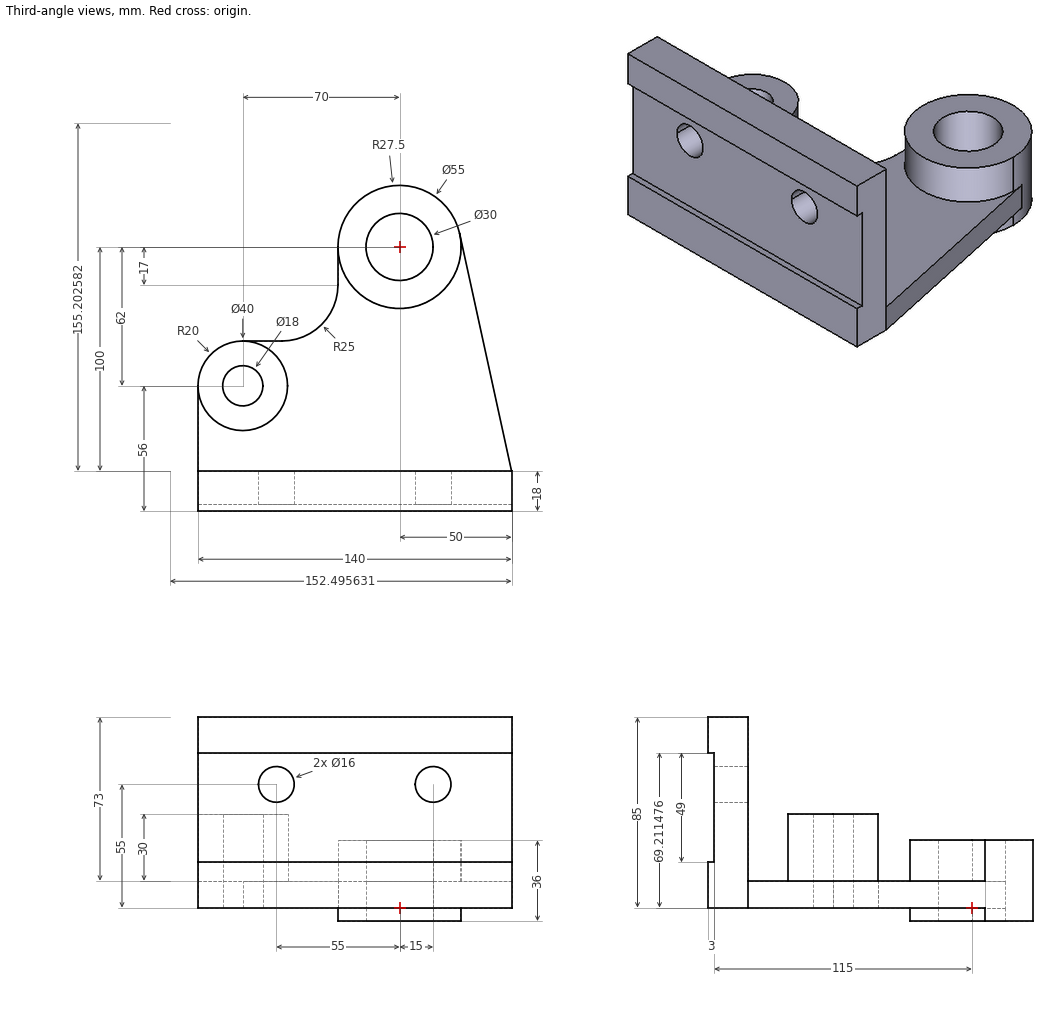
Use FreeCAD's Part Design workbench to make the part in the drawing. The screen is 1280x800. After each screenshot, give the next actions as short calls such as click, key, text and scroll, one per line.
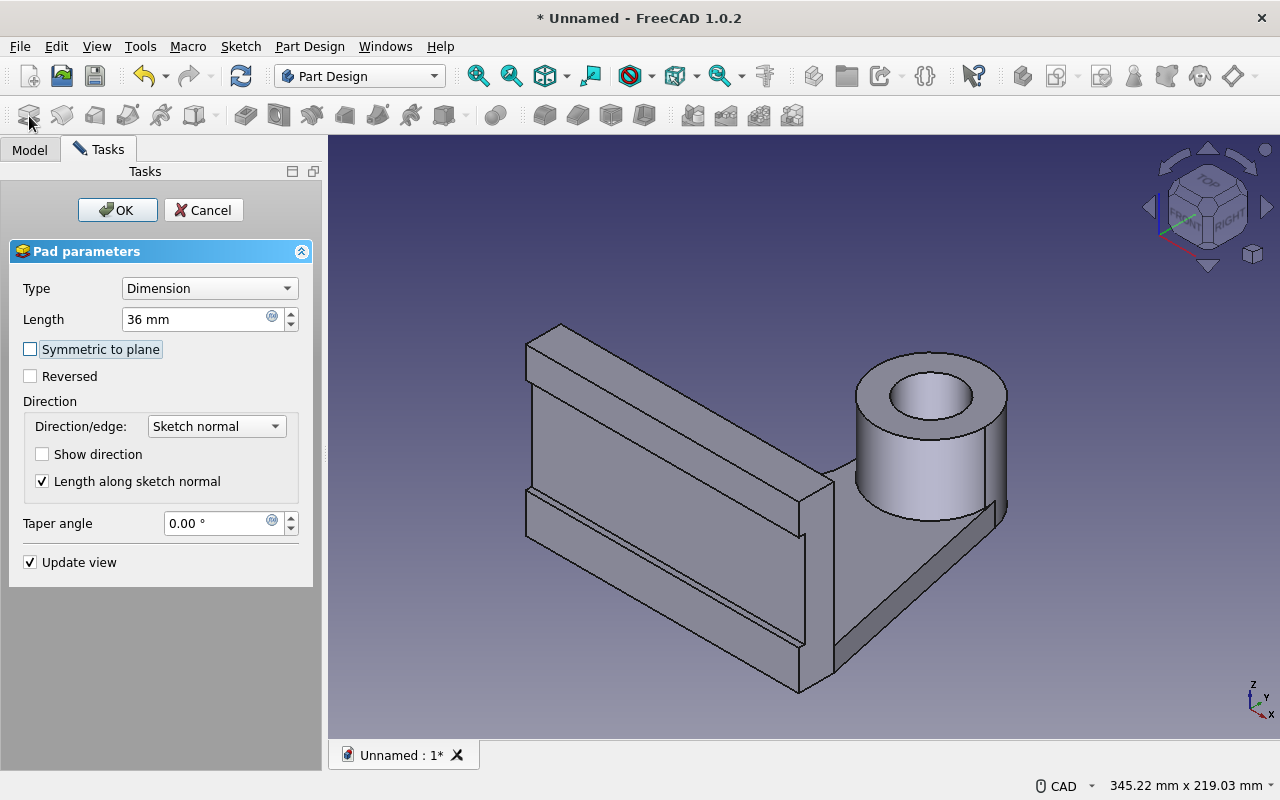
click(31, 349)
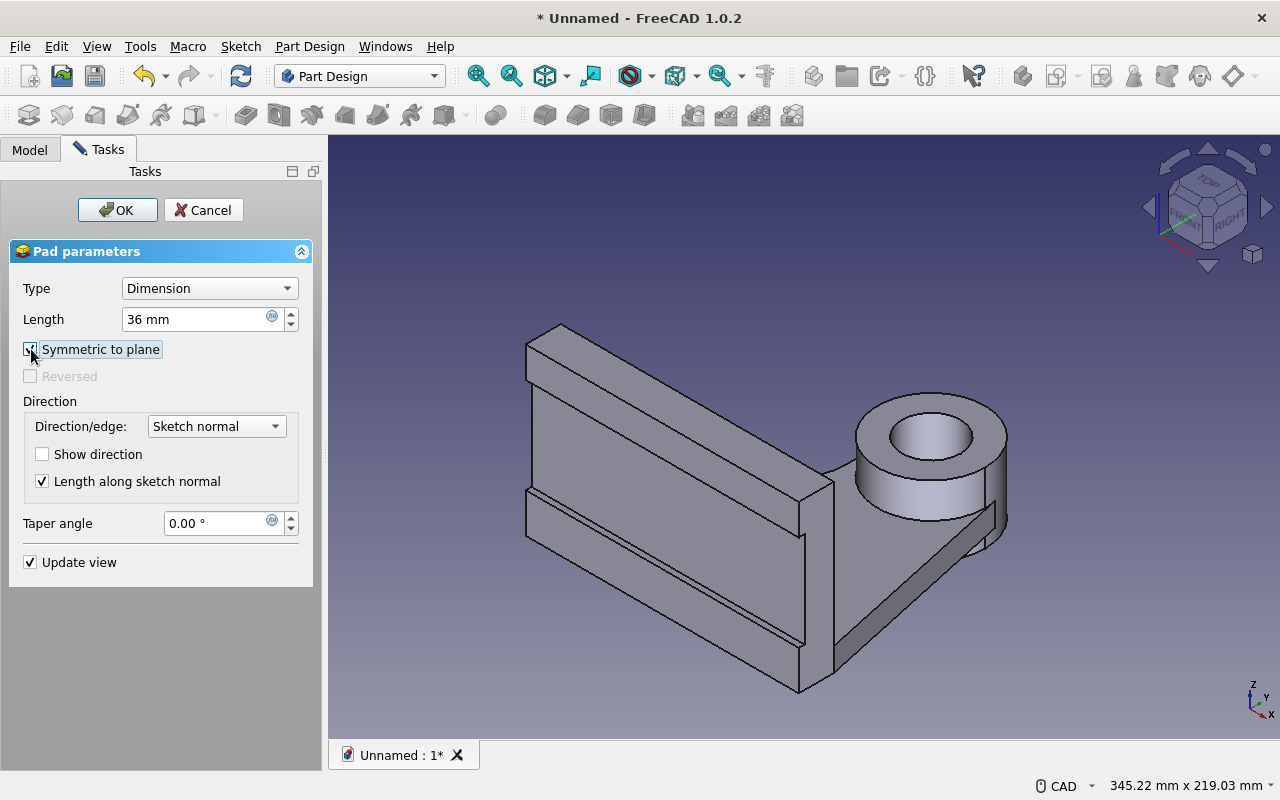
click(118, 210)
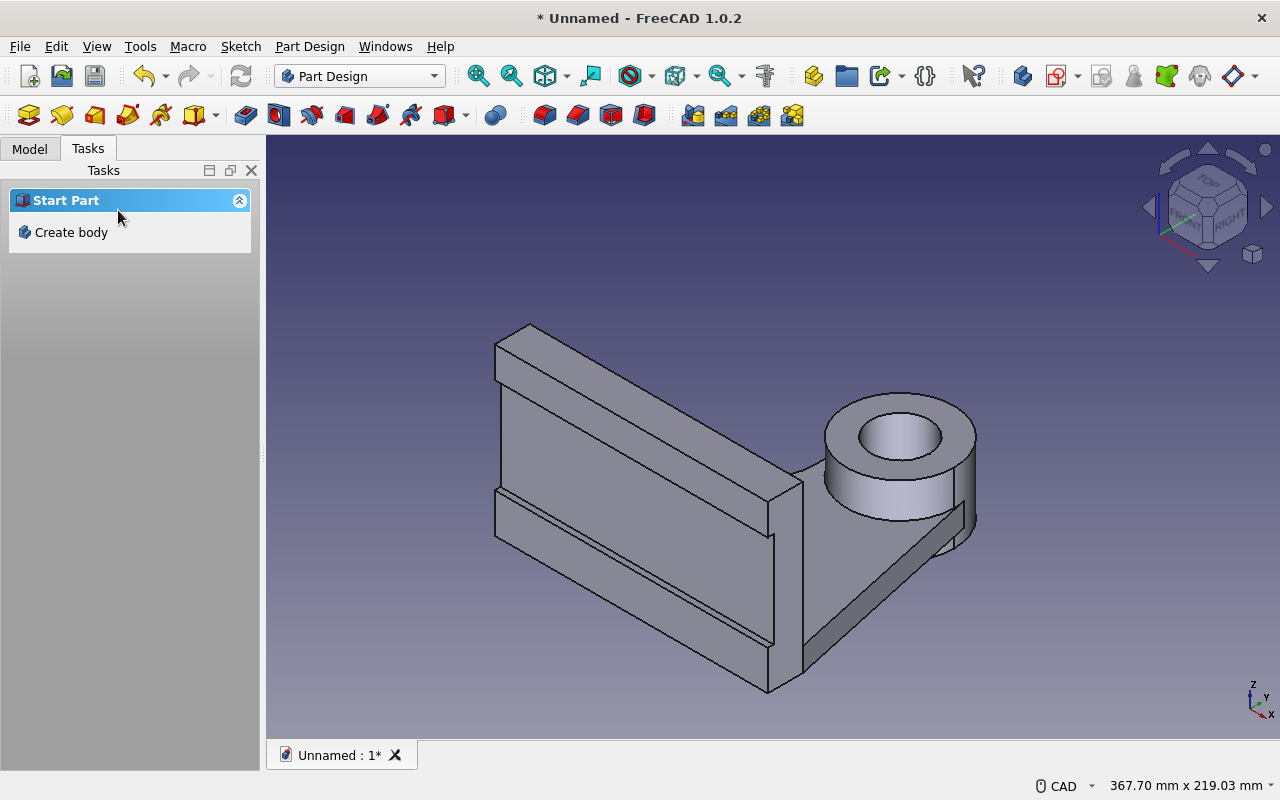
click(818, 569)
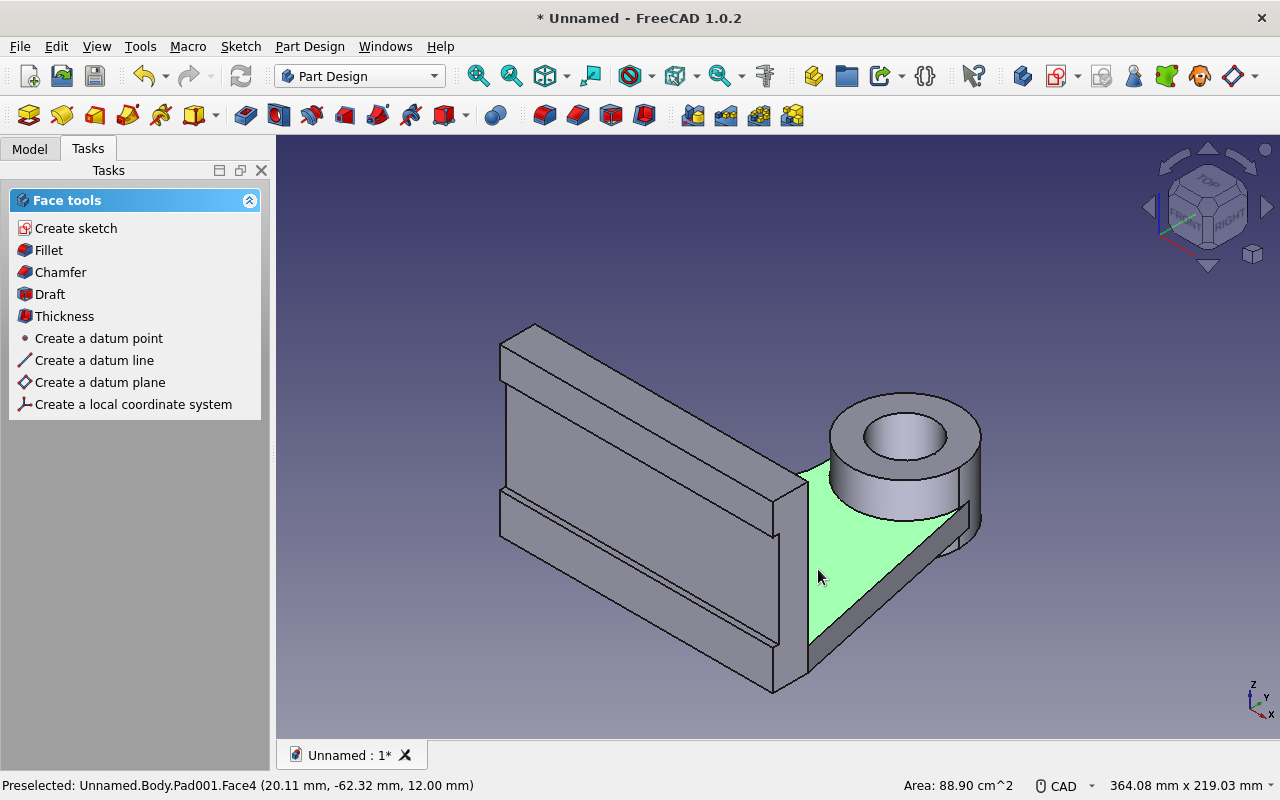
click(1056, 76)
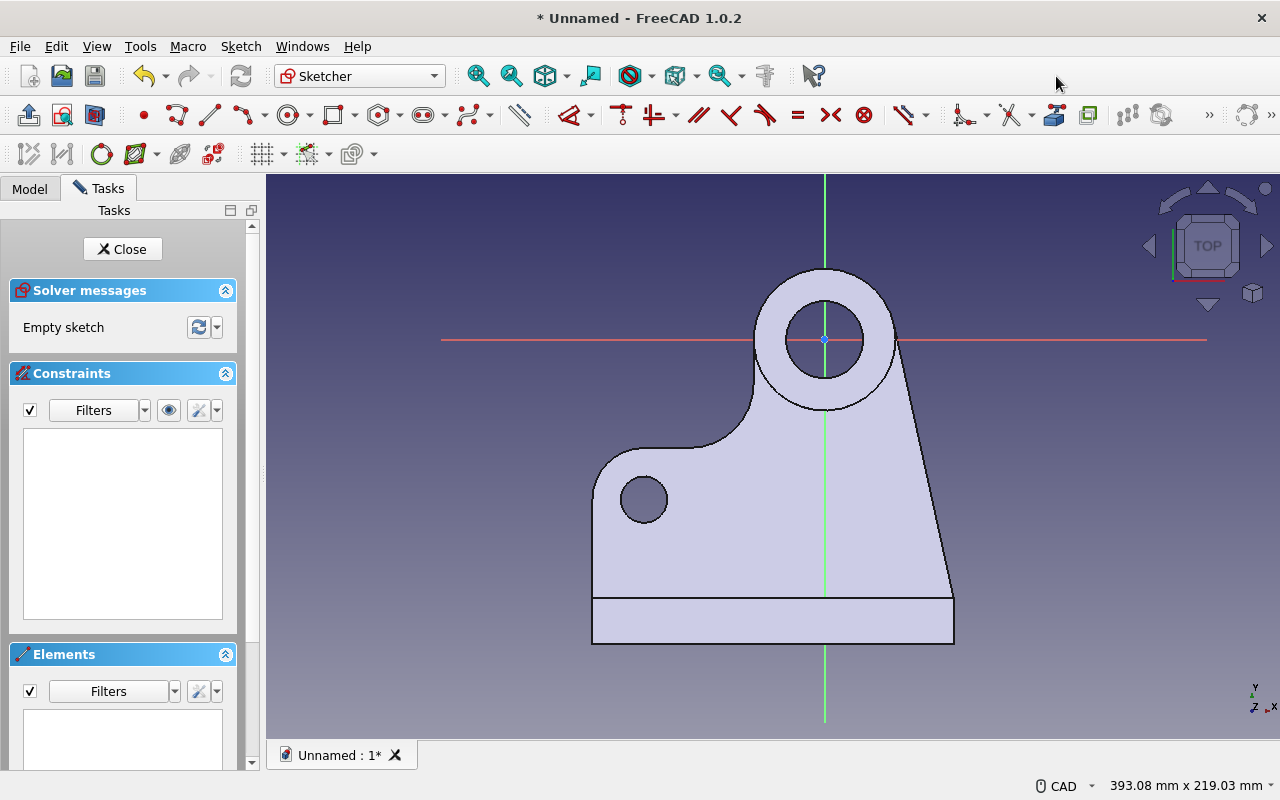
scroll(713, 432, up, 3)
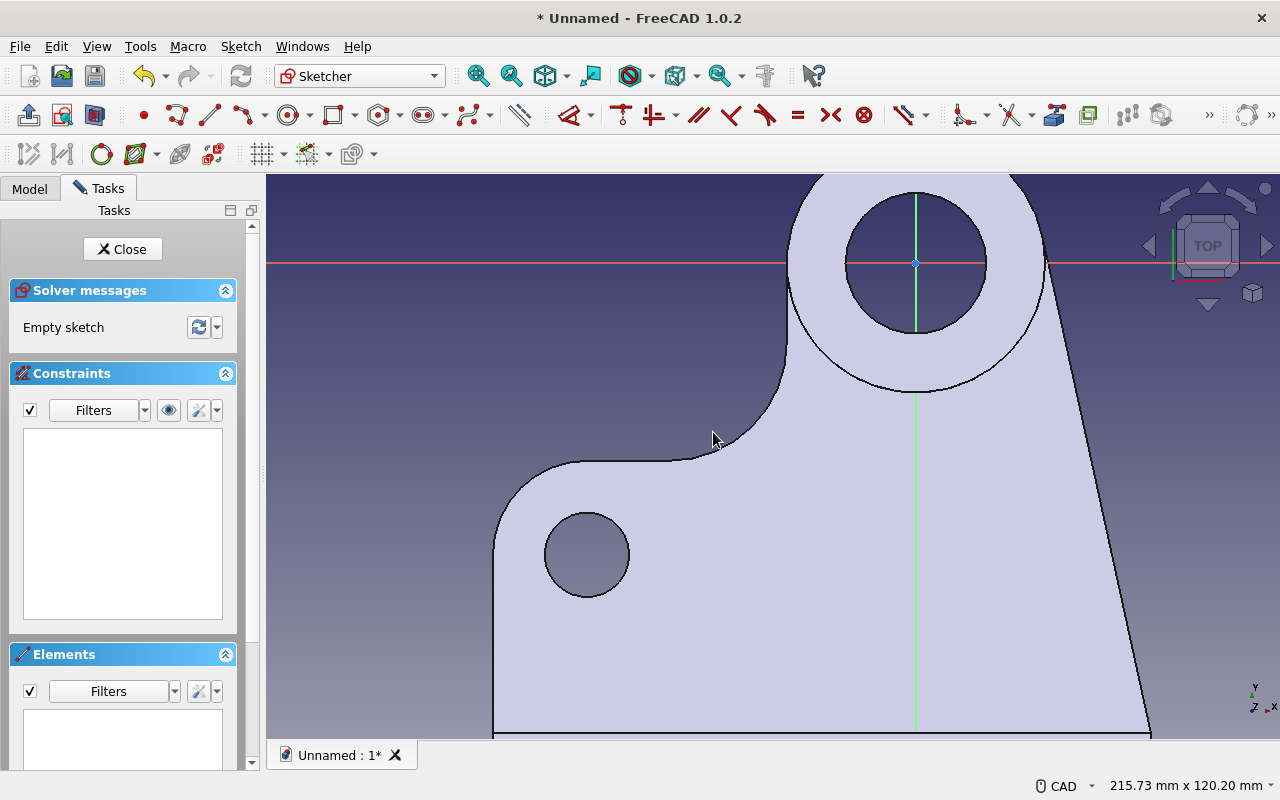
click(288, 116)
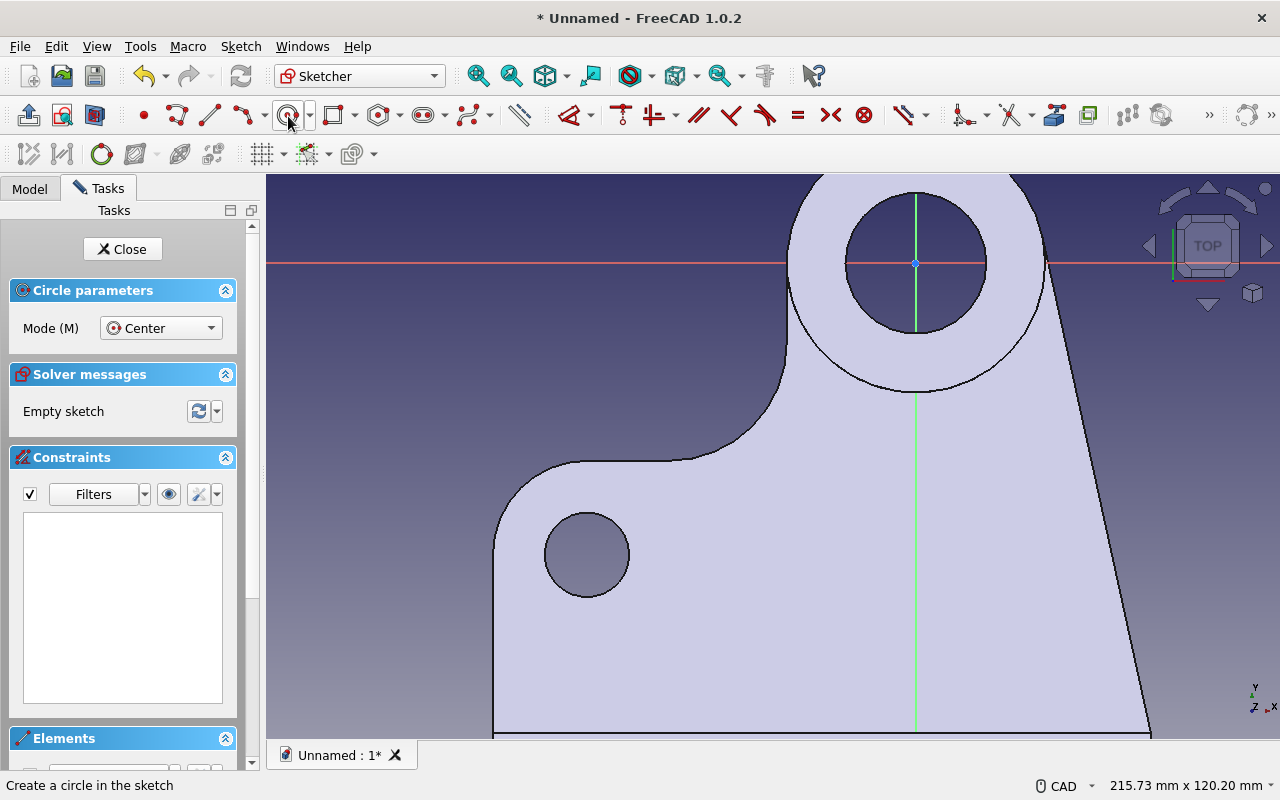
click(587, 555)
click(653, 488)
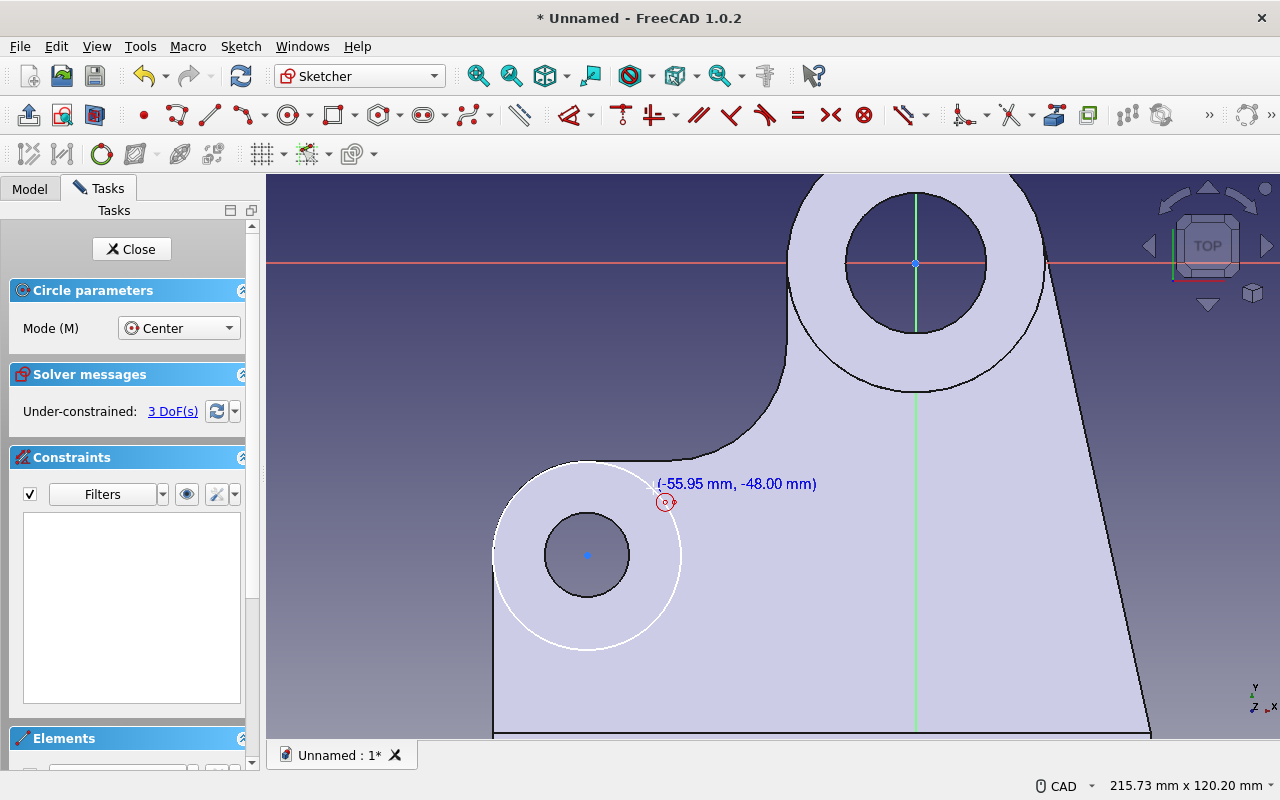
click(587, 556)
click(617, 525)
key(Escape)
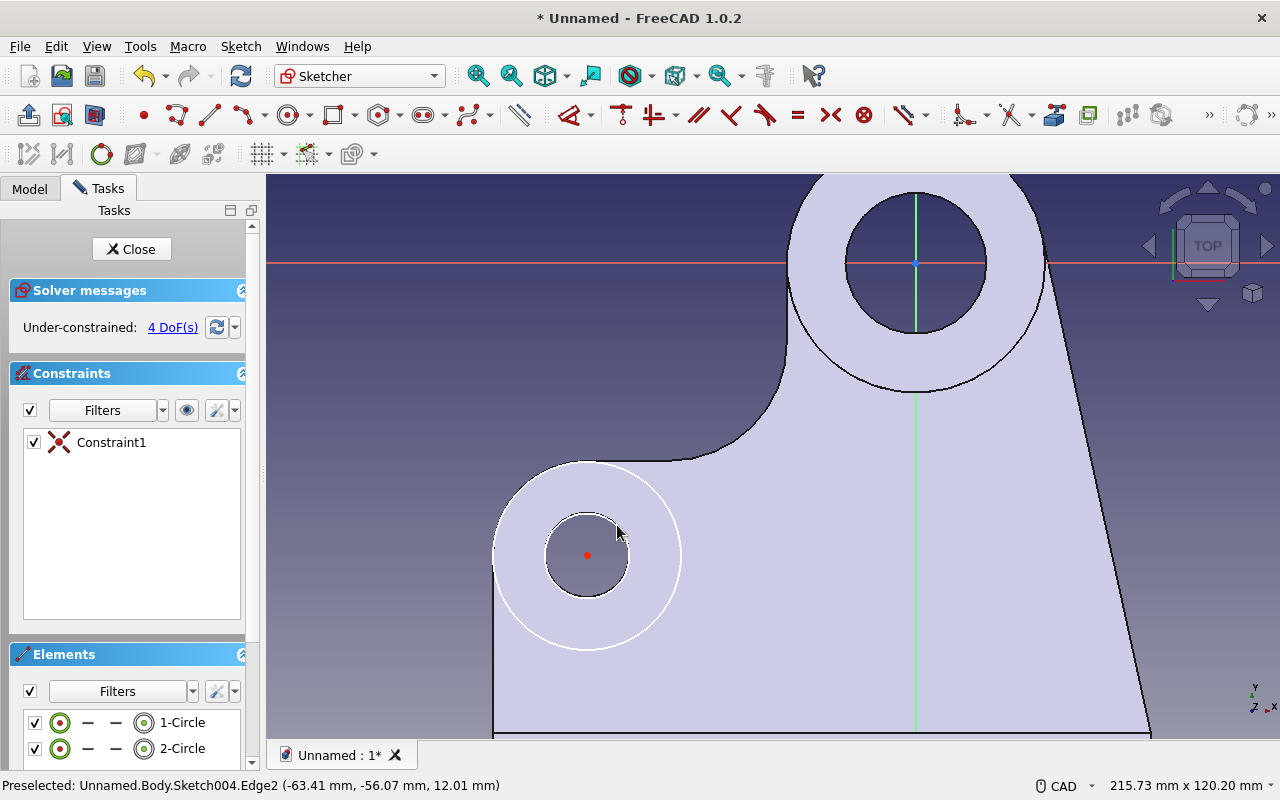
click(568, 116)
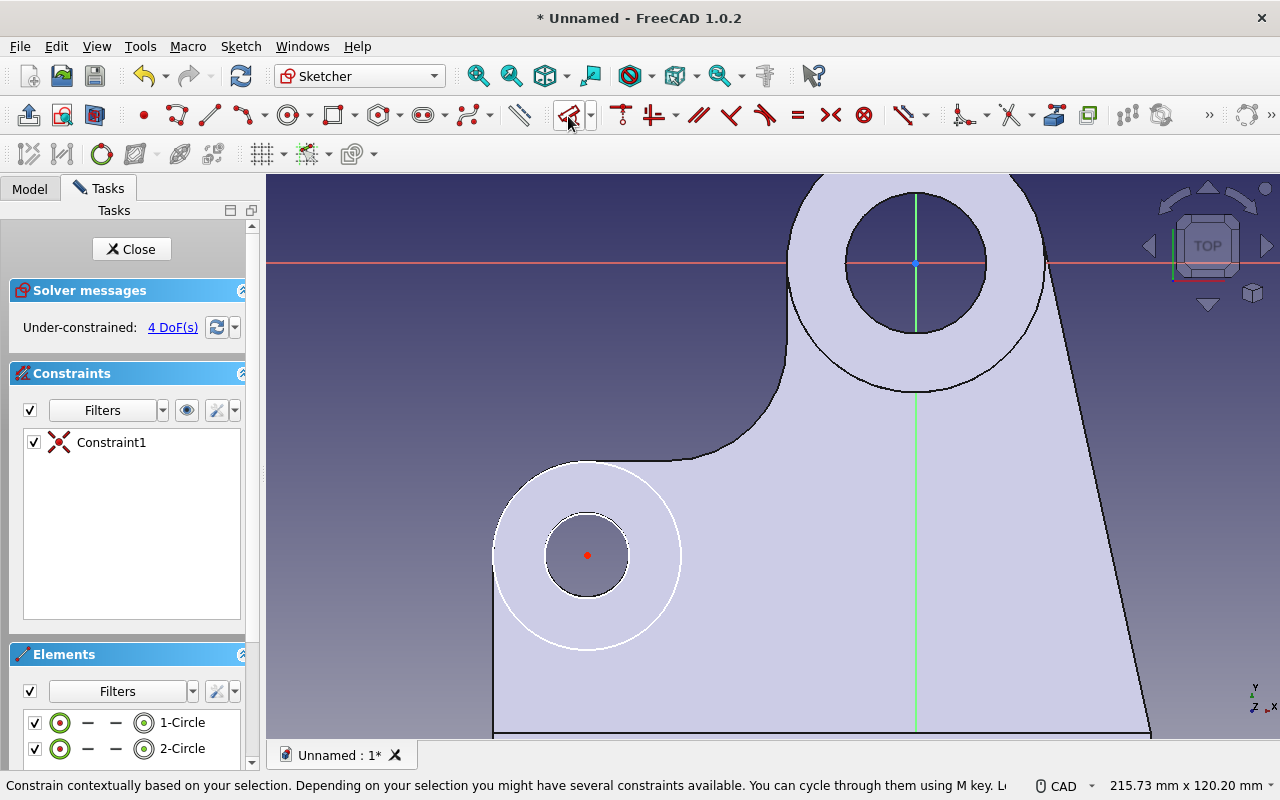
click(653, 489)
click(675, 466)